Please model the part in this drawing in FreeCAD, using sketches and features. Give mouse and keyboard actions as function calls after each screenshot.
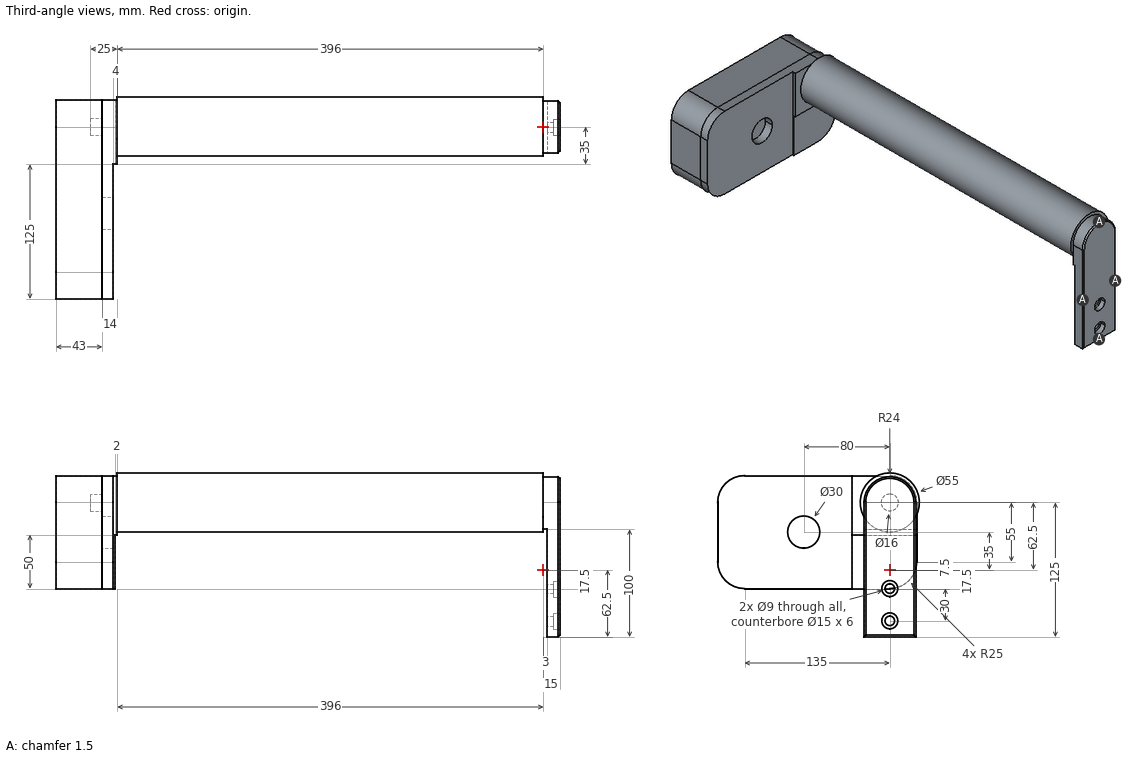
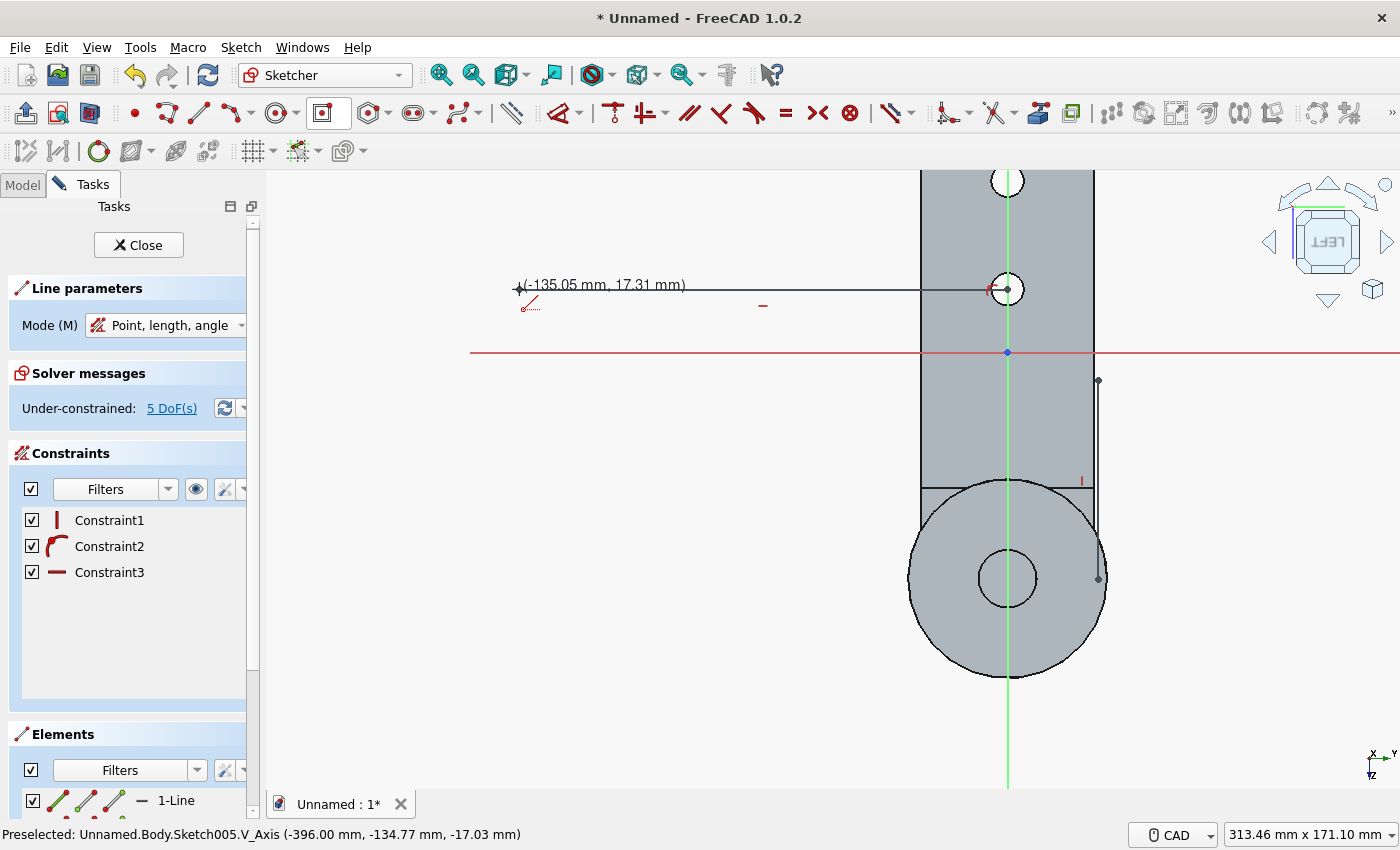
click(429, 380)
click(429, 579)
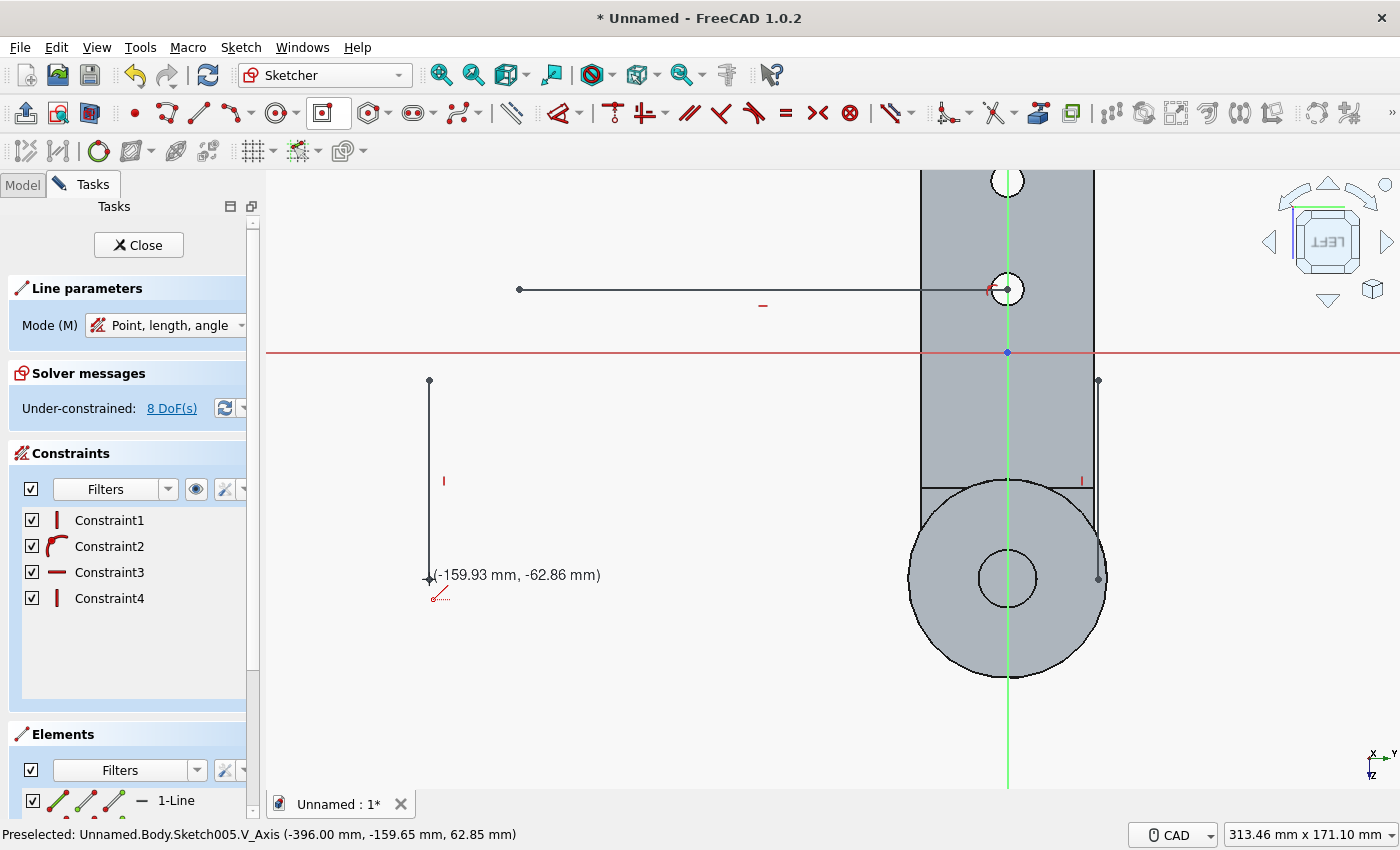
click(519, 669)
click(1008, 669)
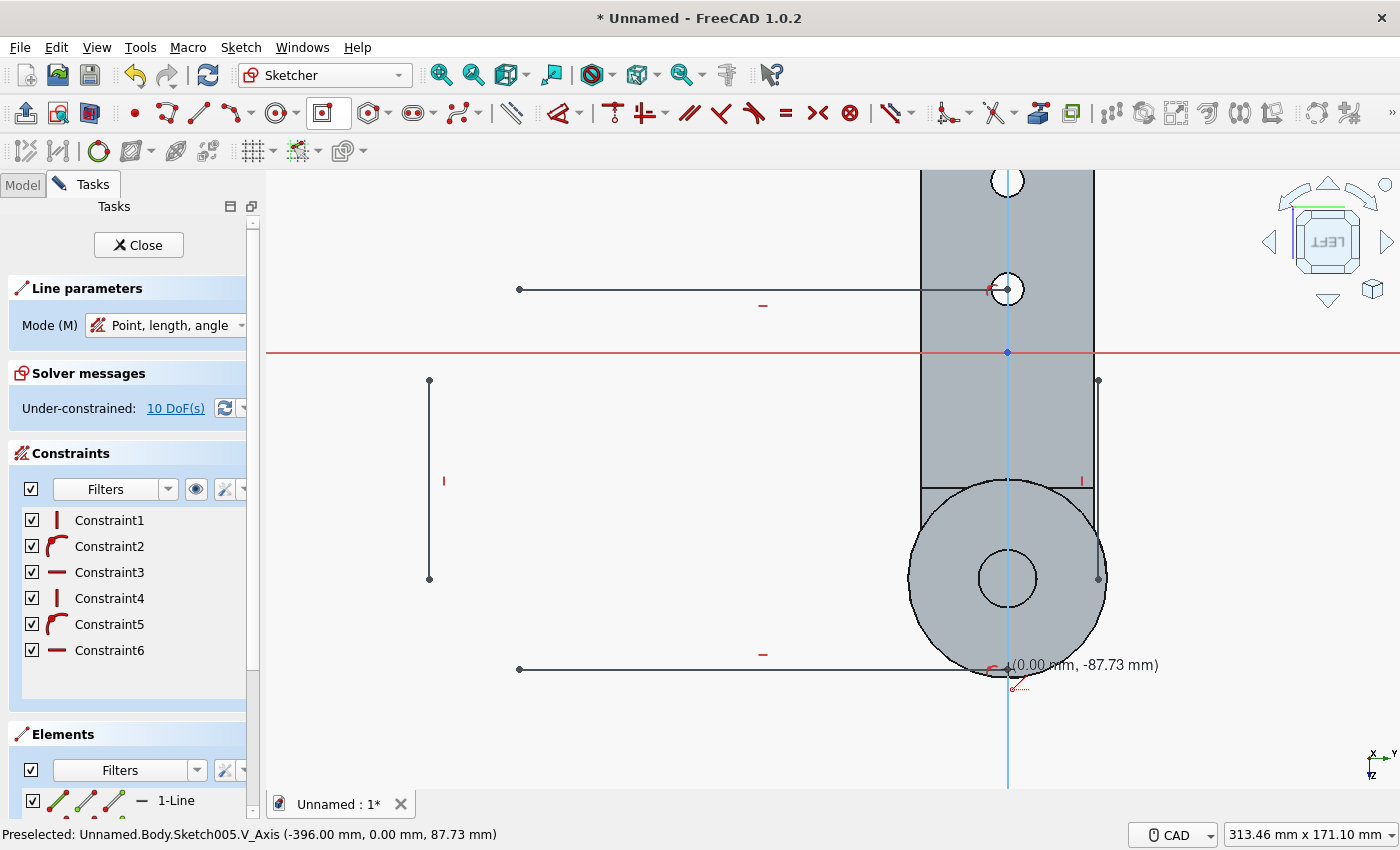
key(g)
key(3)
key(a)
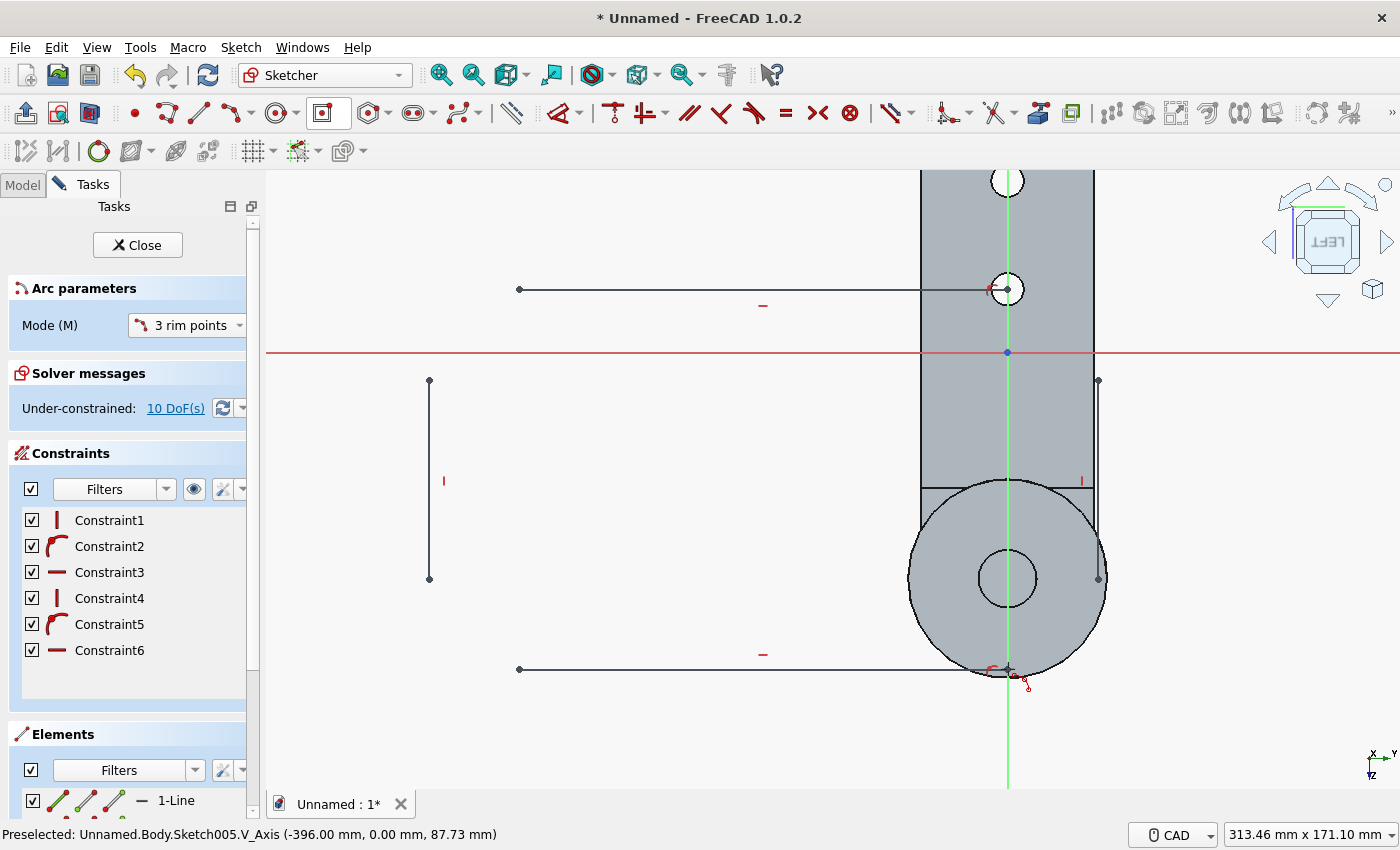
click(1098, 381)
click(1008, 290)
click(1072, 316)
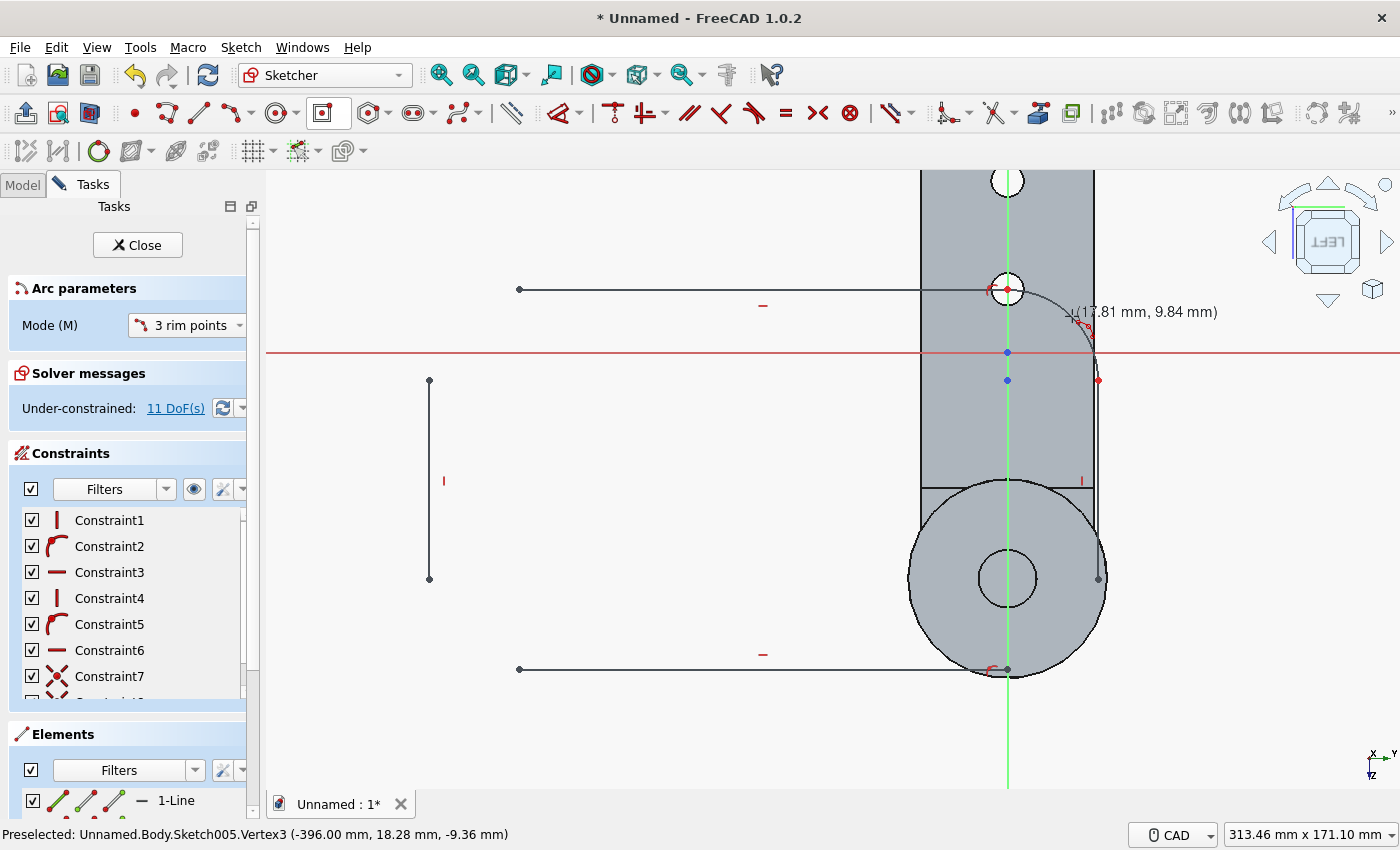
click(519, 290)
click(429, 381)
click(455, 316)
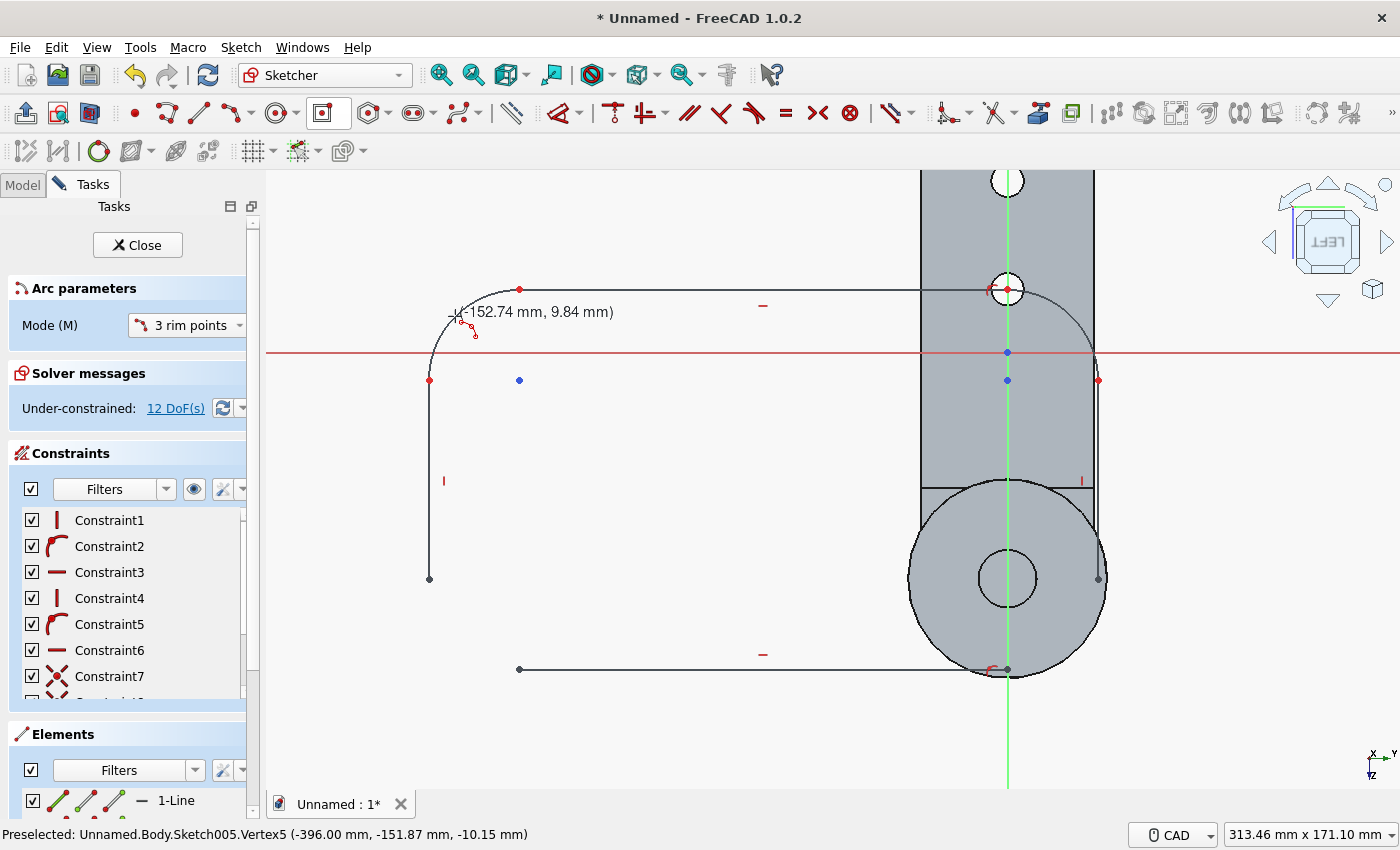
click(429, 580)
click(519, 670)
click(455, 643)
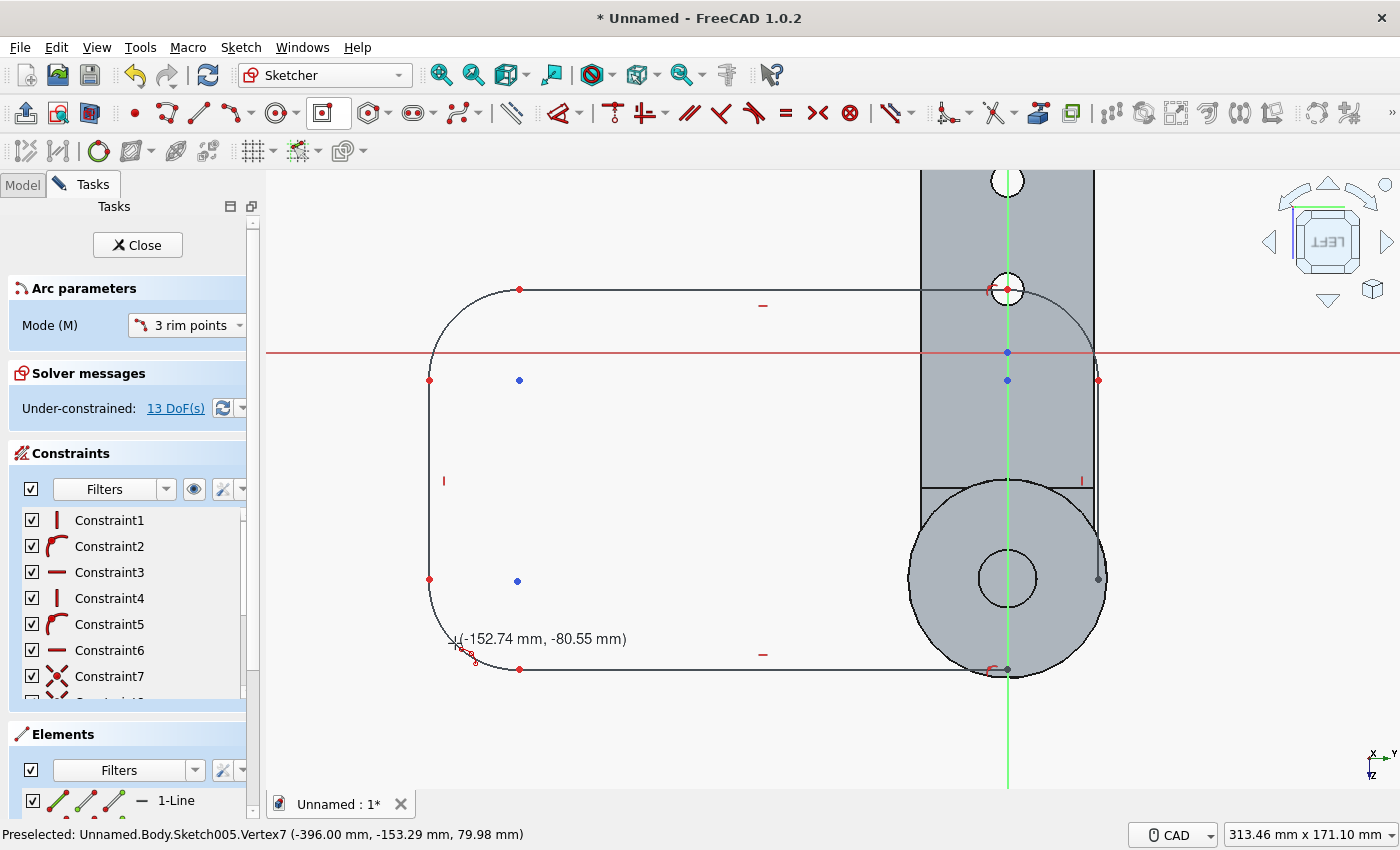
click(1008, 670)
click(1098, 580)
click(1072, 643)
key(Escape)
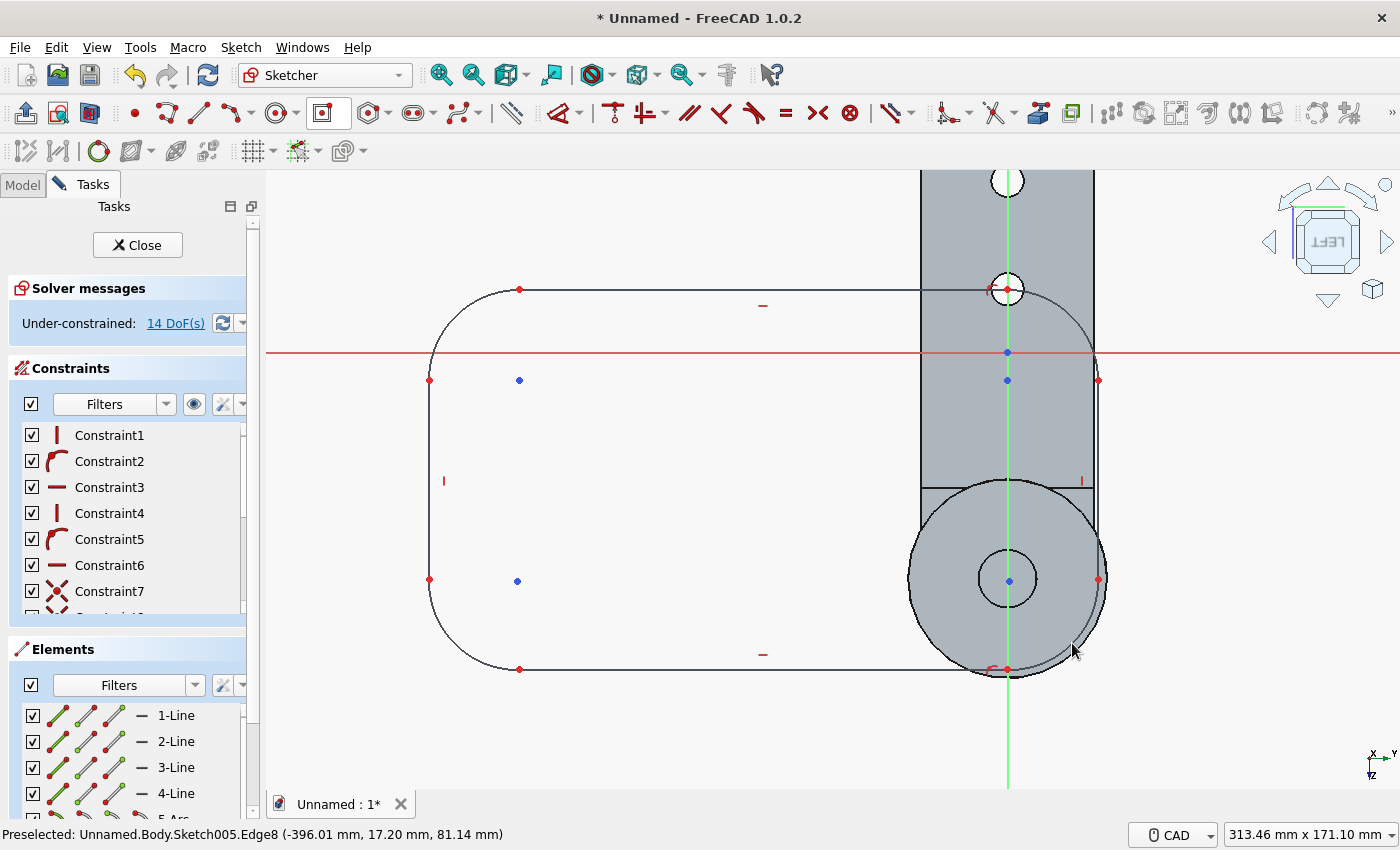
click(1098, 520)